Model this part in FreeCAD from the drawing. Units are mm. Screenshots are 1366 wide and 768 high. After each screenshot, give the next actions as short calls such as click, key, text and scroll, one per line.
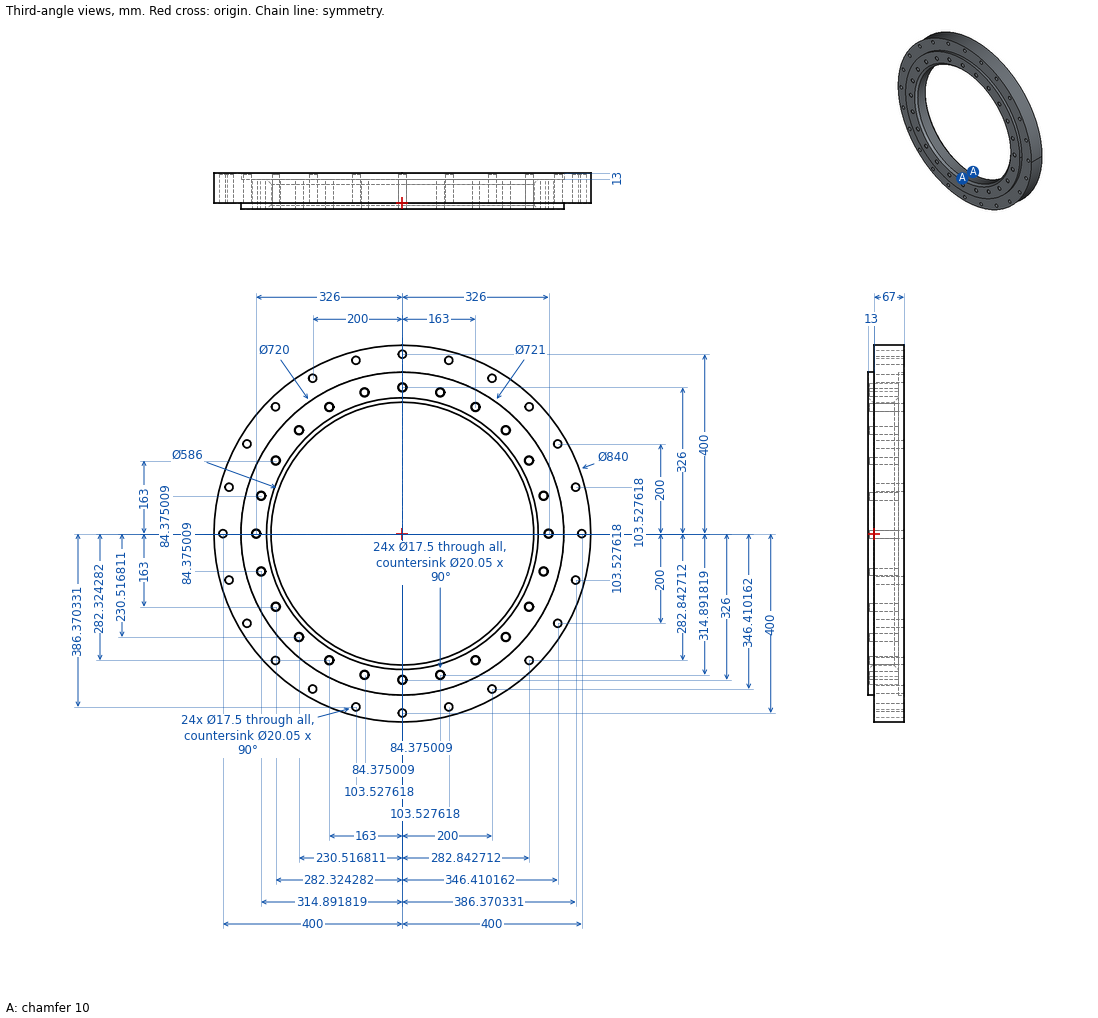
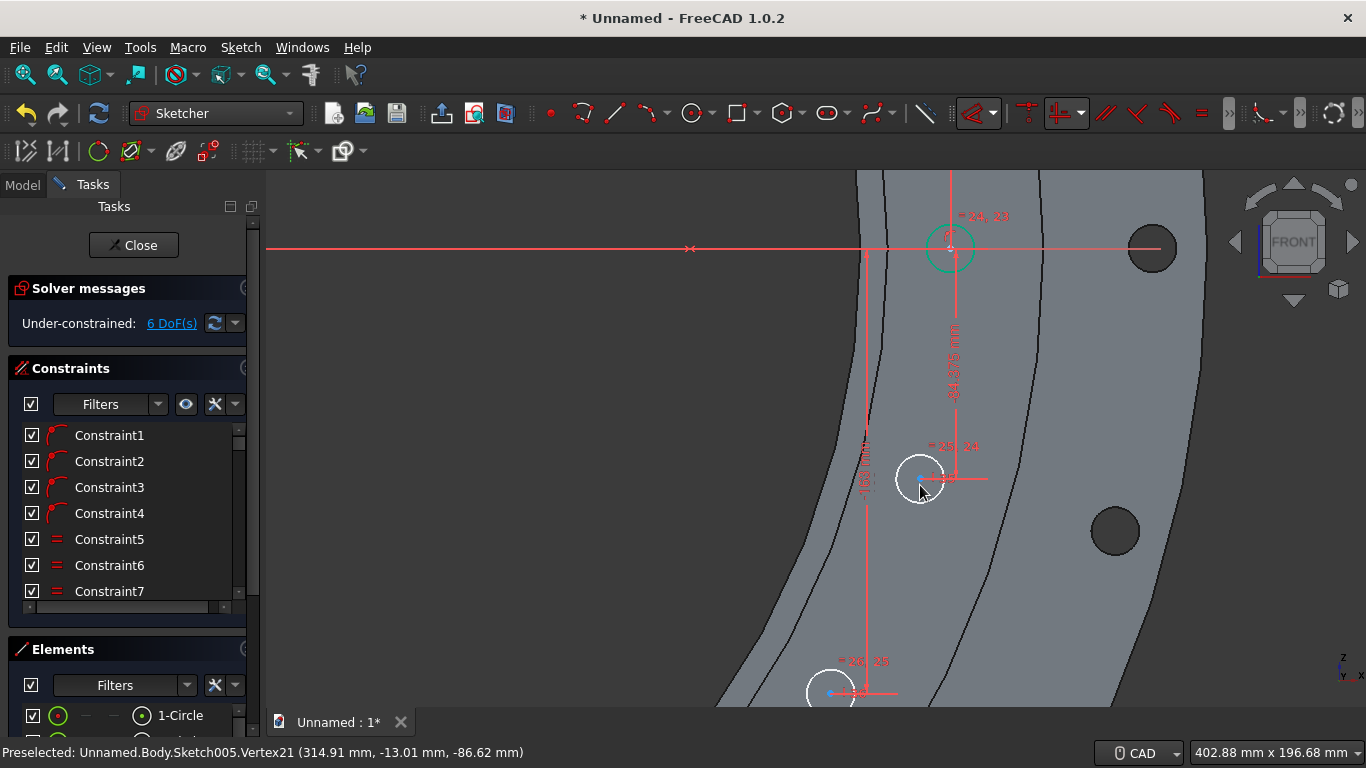
scroll(921, 487, down, 8)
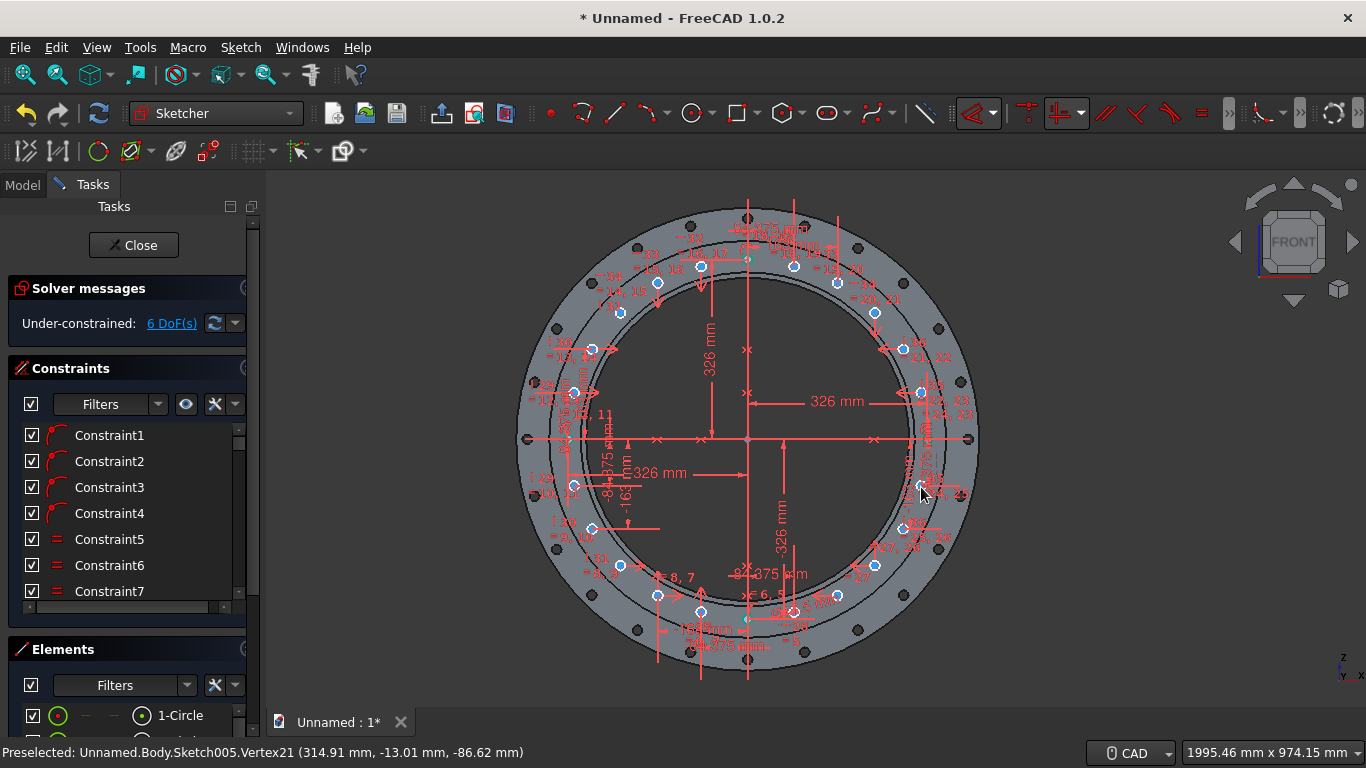
click(794, 612)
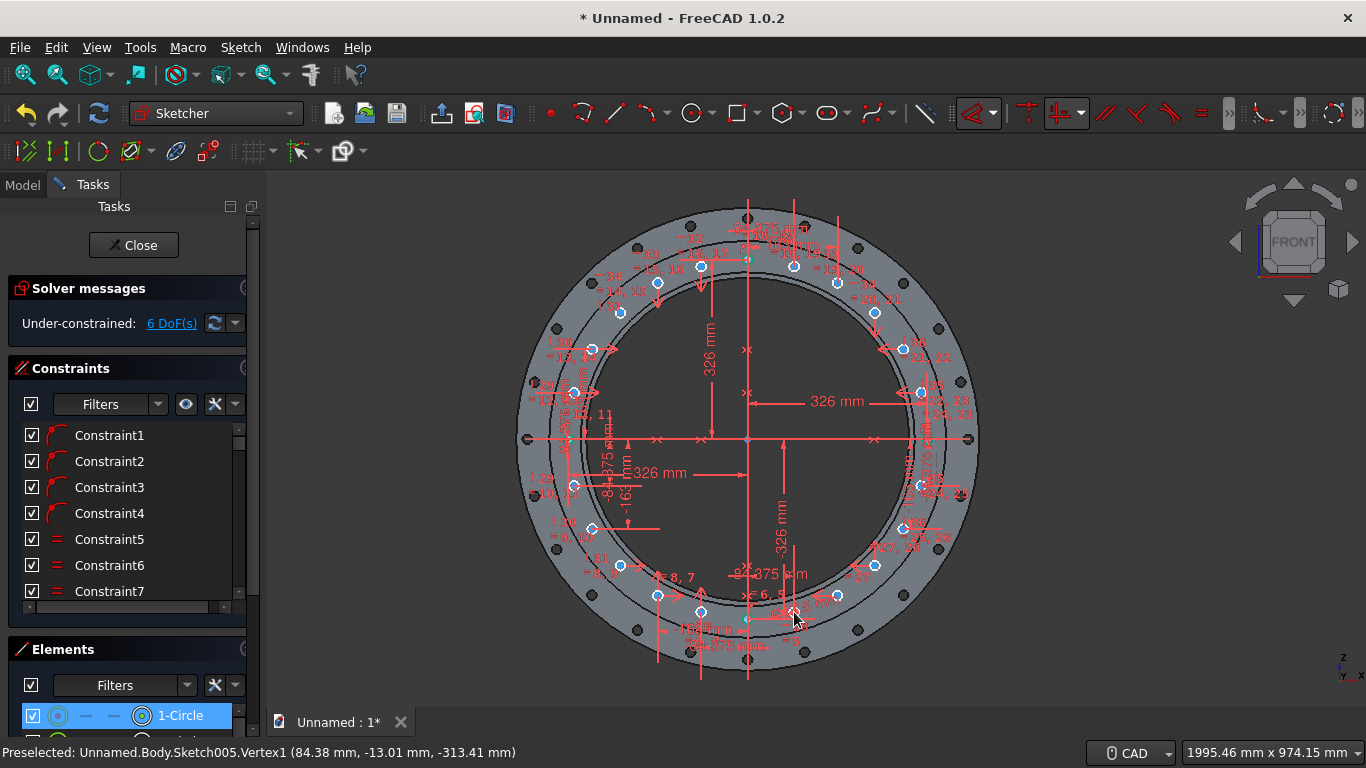
key(i)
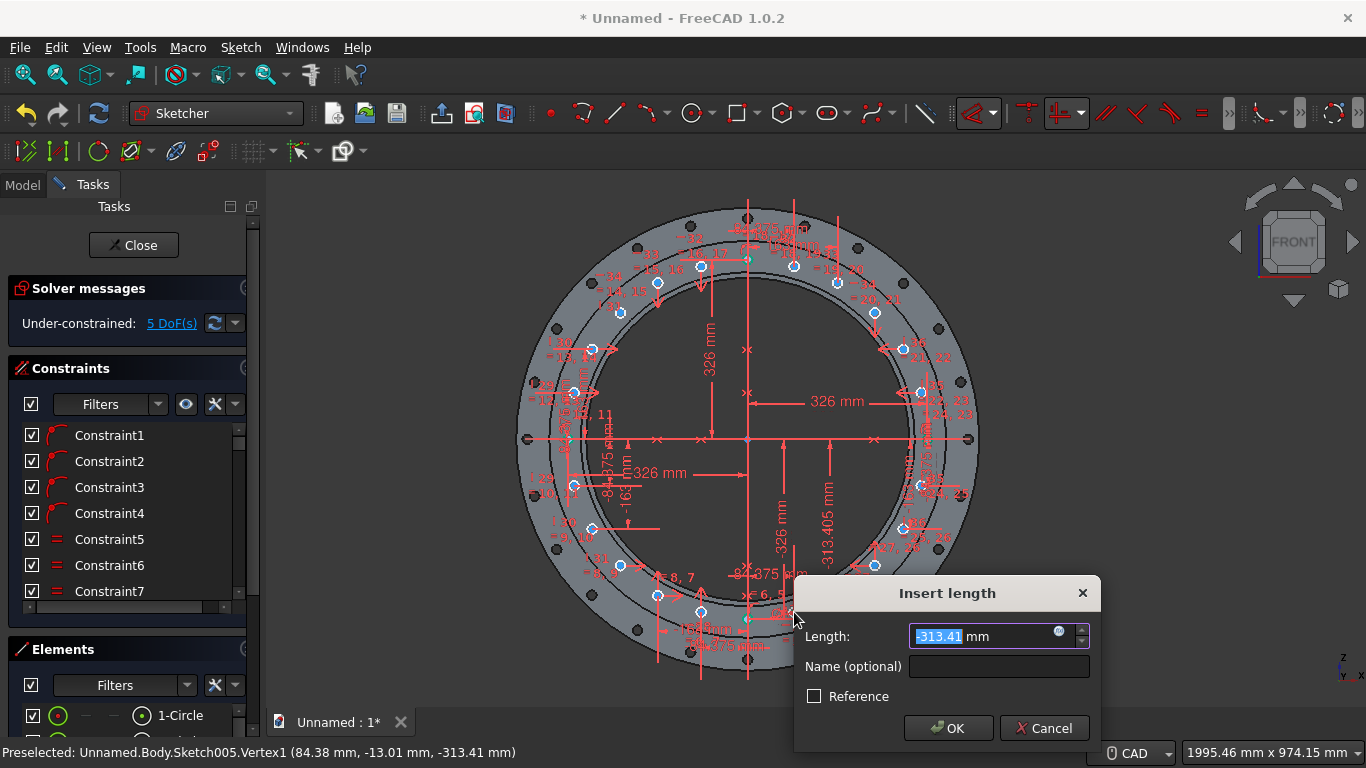
text(-314.891819)
key(Return)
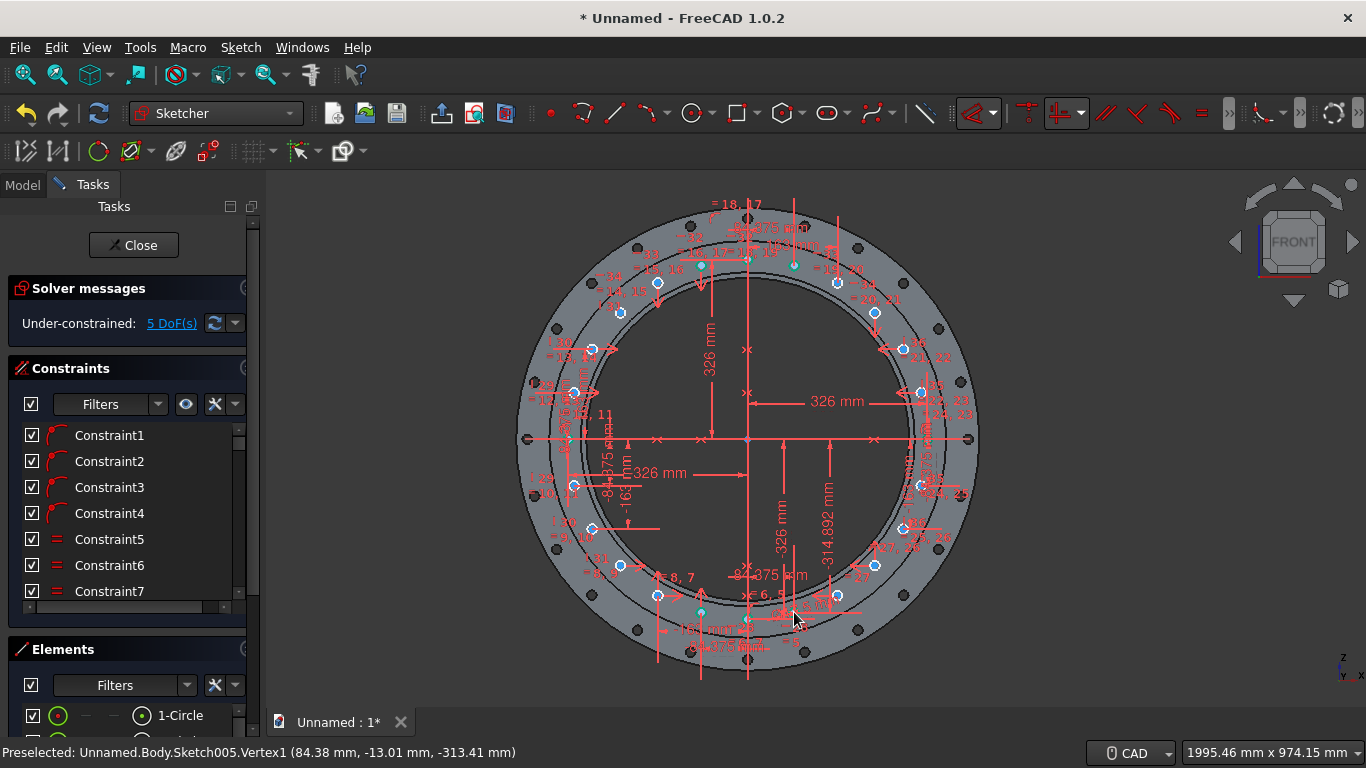
click(658, 596)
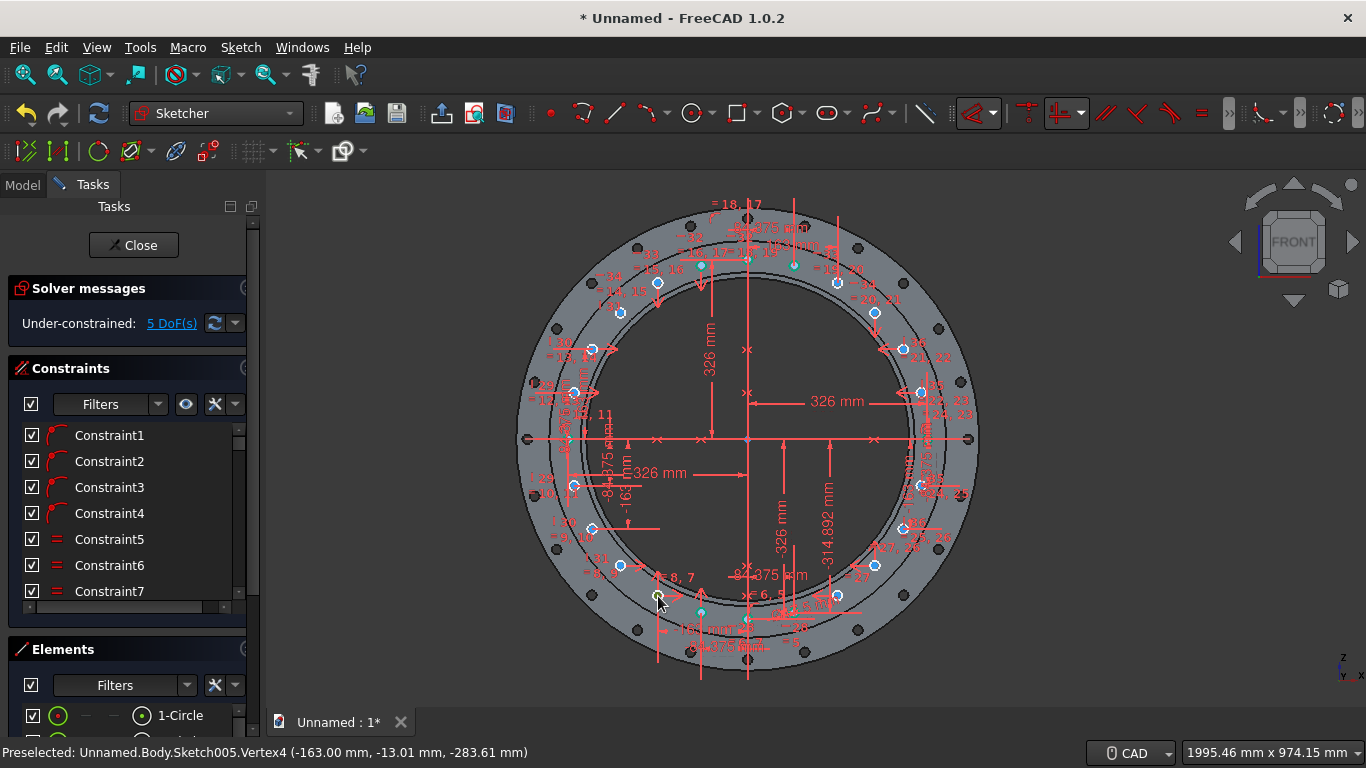
click(996, 114)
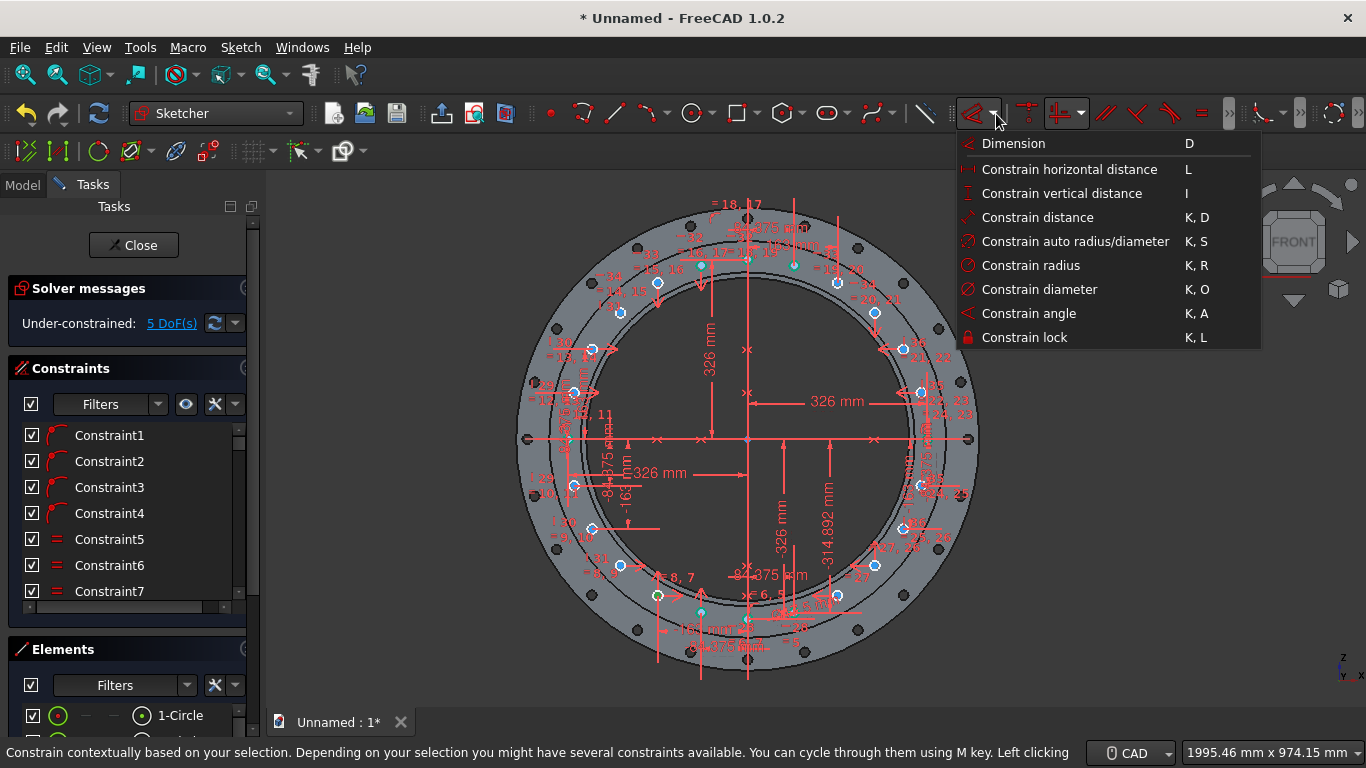
click(1109, 193)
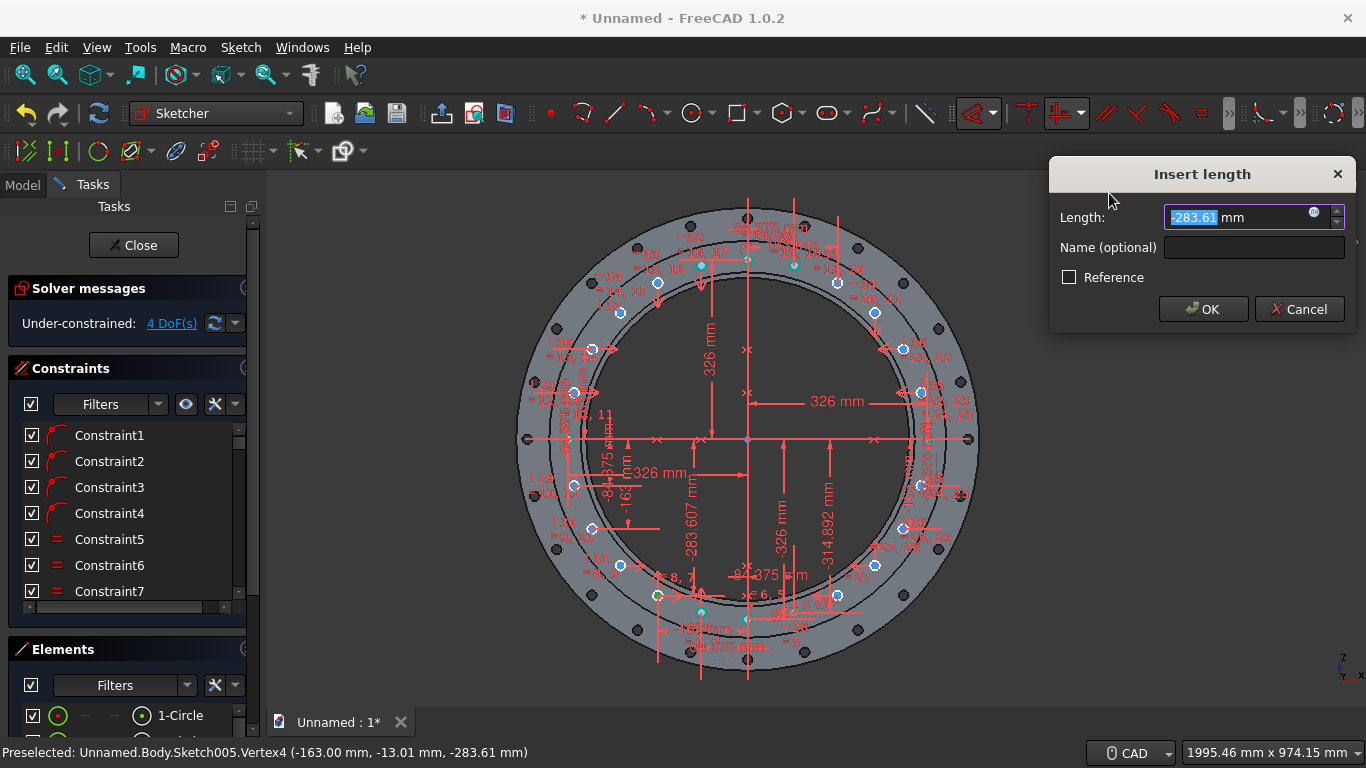
text(-282.324282)
key(Return)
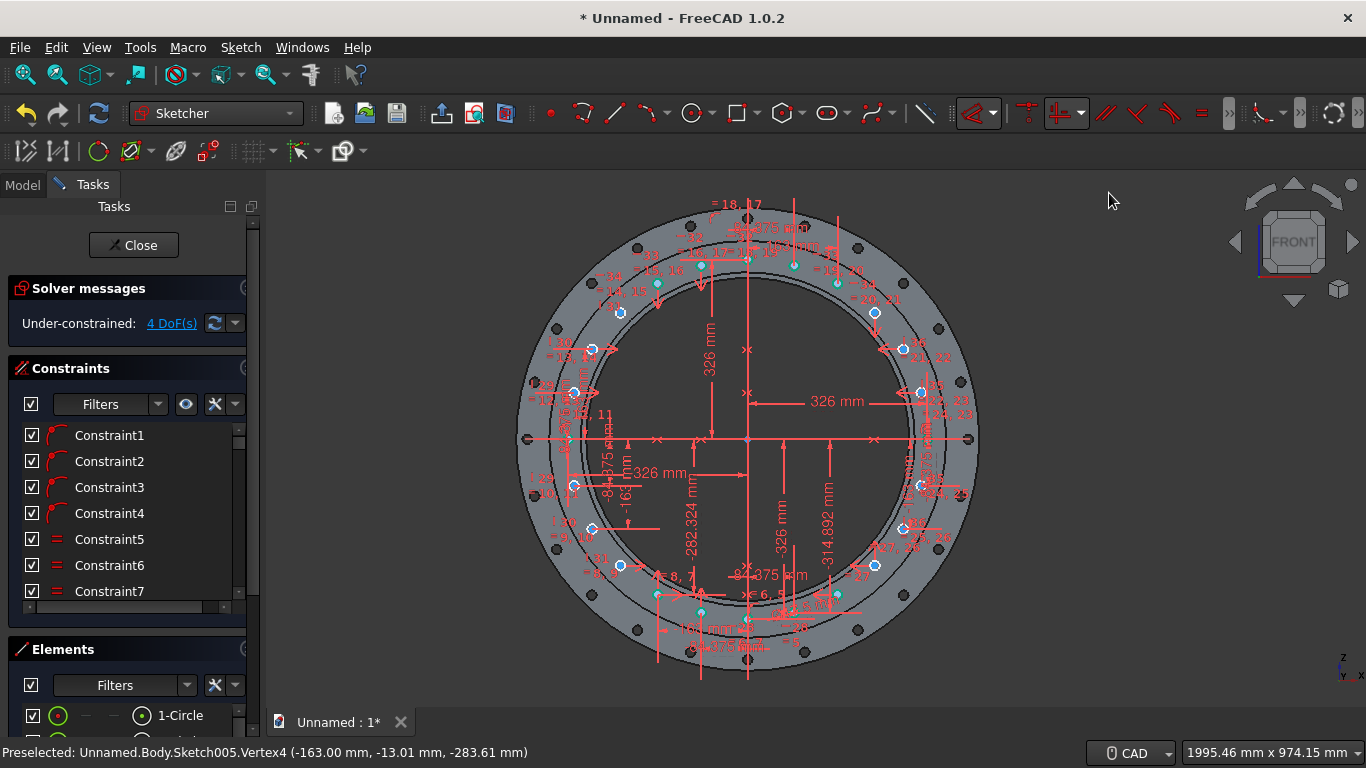
click(620, 566)